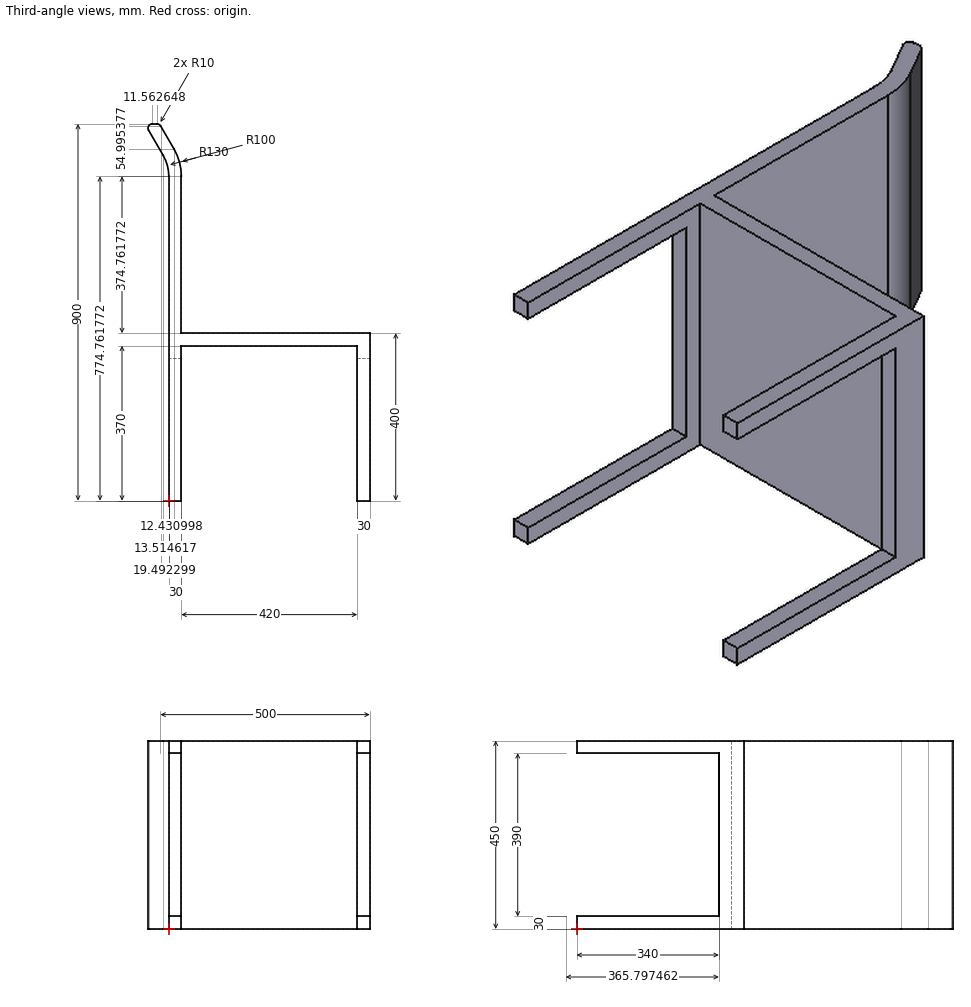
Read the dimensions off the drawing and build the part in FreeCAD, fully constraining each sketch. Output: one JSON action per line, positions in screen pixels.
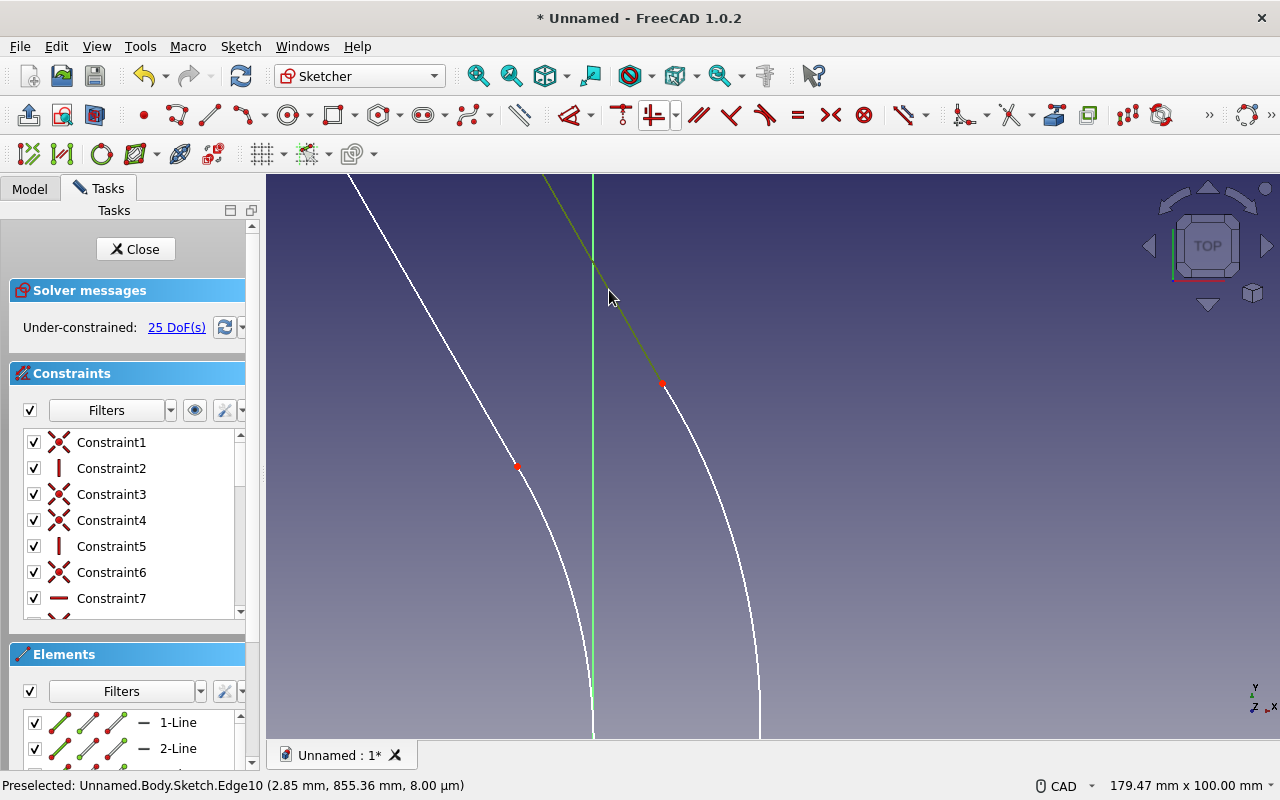
{"action": "scroll", "coordinate": [616, 286], "scroll_direction": "down", "scroll_amount": 13}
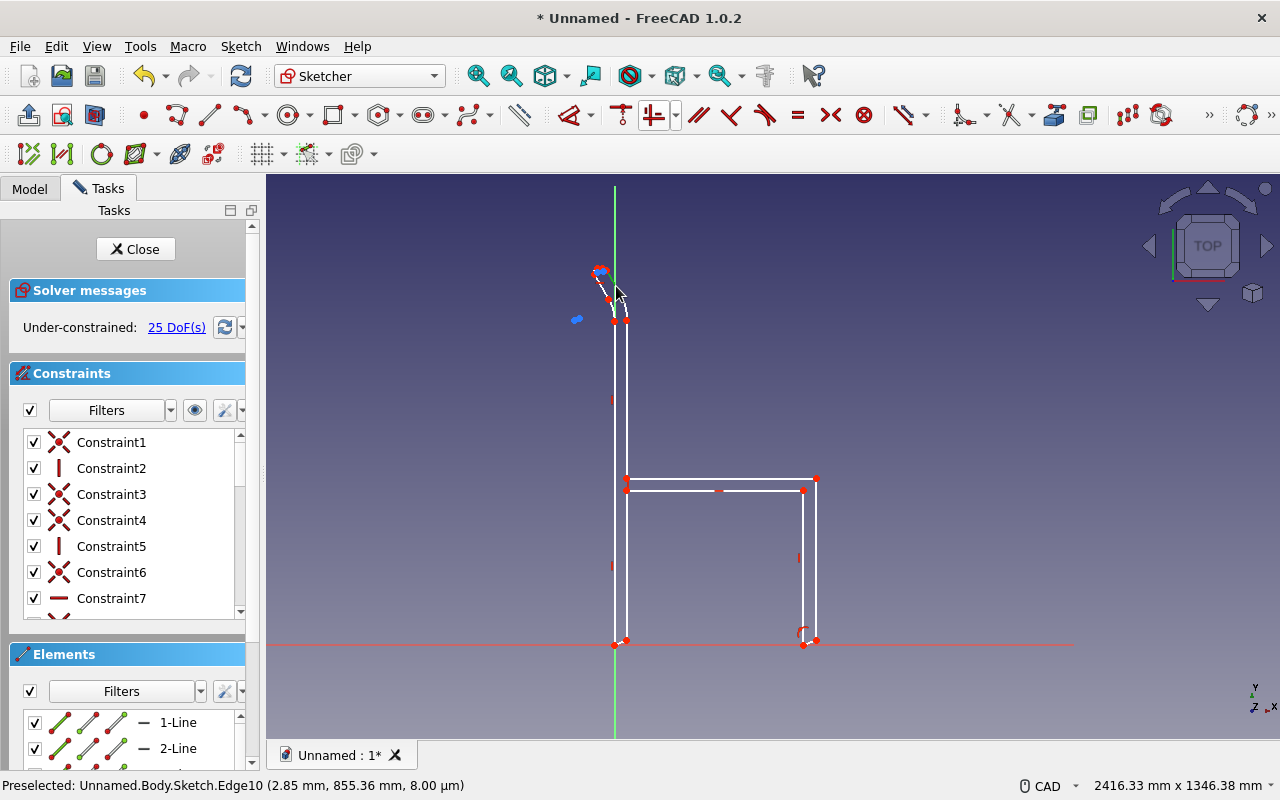
{"action": "scroll", "coordinate": [606, 269], "scroll_direction": "up", "scroll_amount": 12}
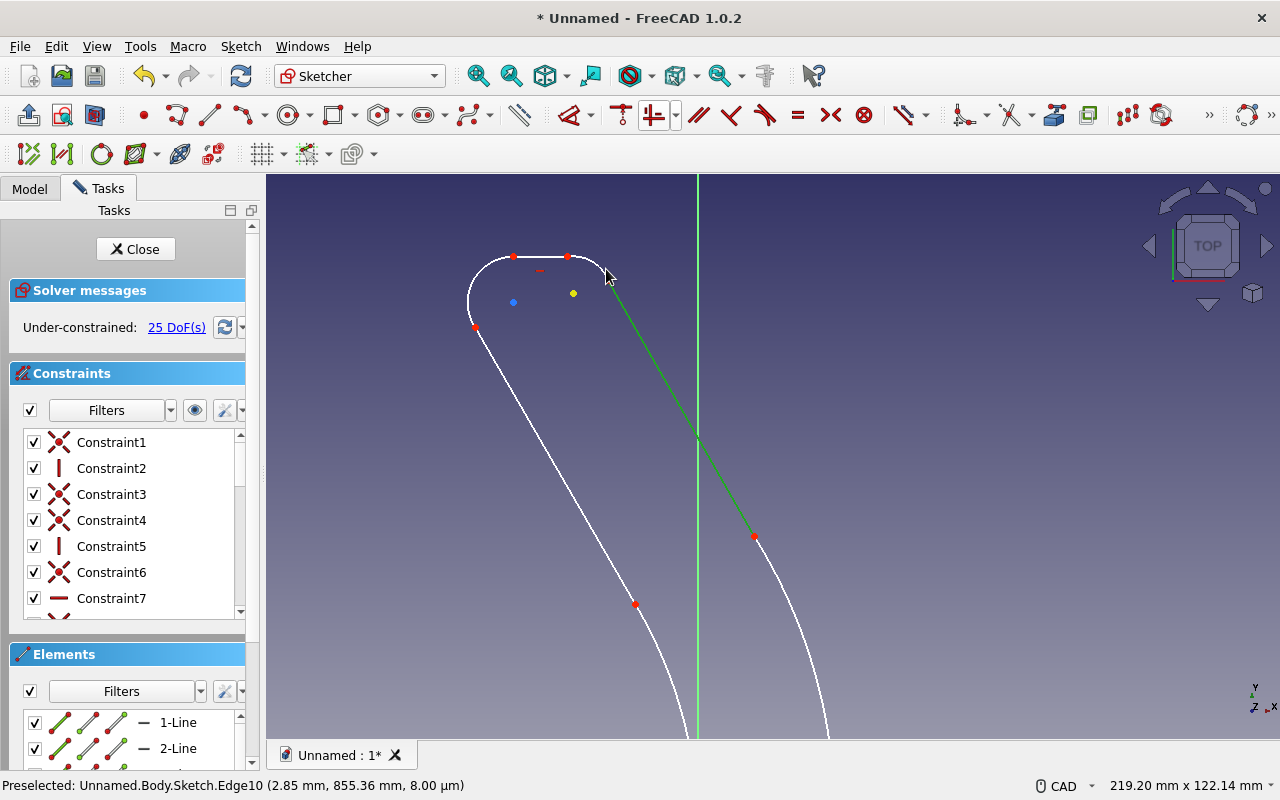
{"action": "left_click", "coordinate": [600, 268]}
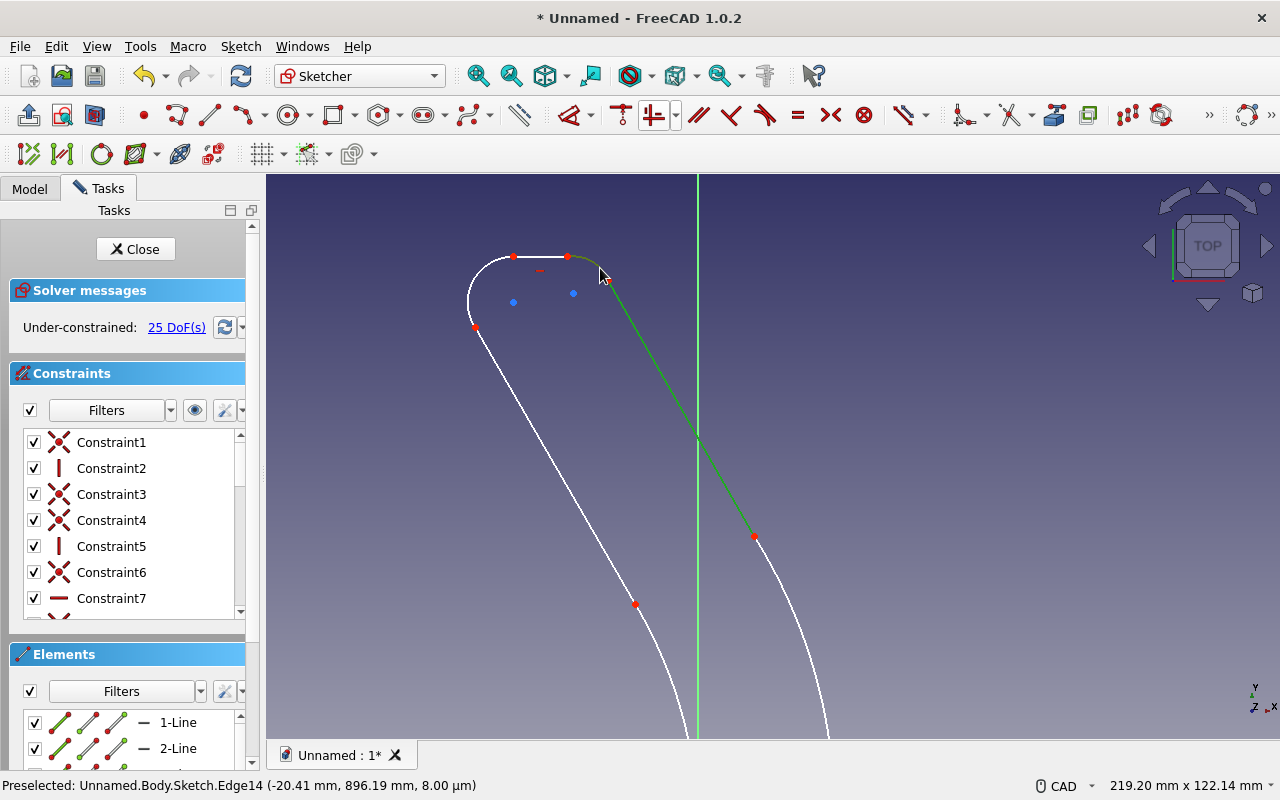
{"action": "left_click", "coordinate": [765, 116]}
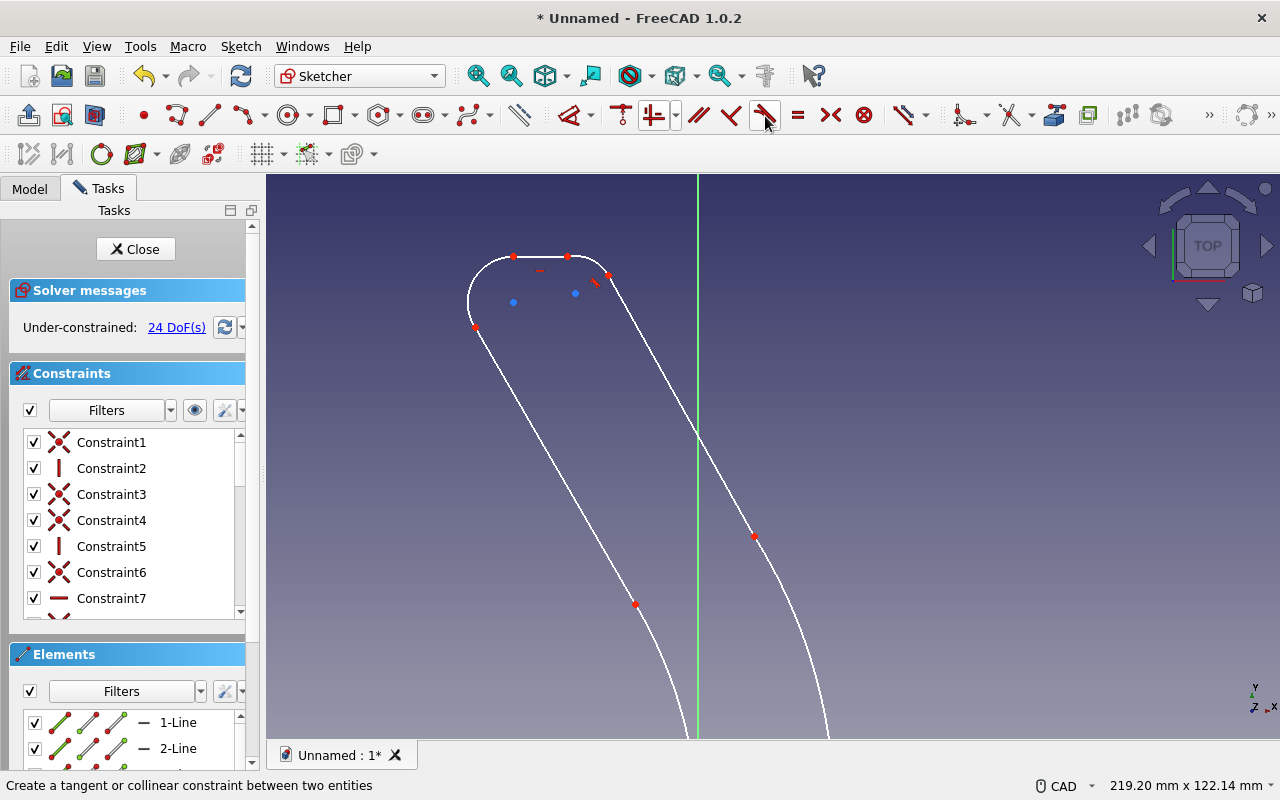
{"action": "left_click", "coordinate": [551, 257]}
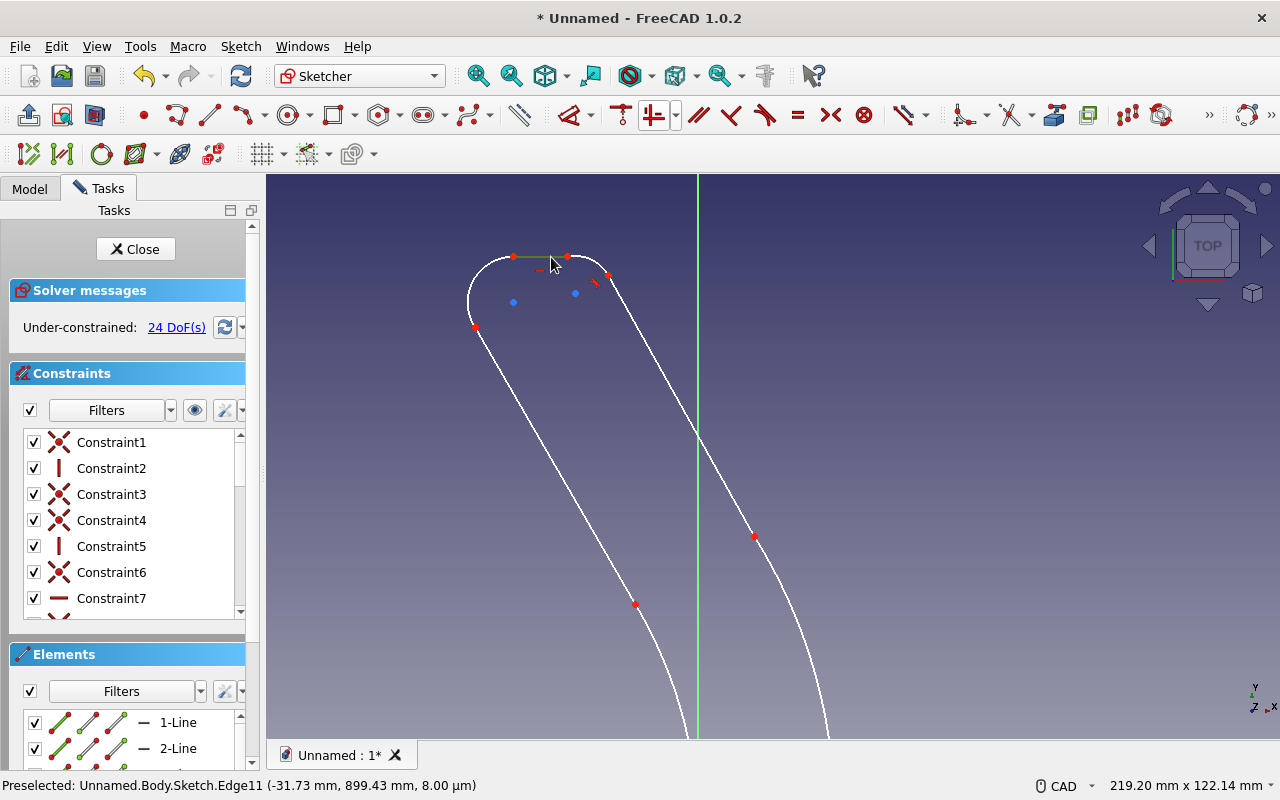
{"action": "left_click", "coordinate": [599, 264]}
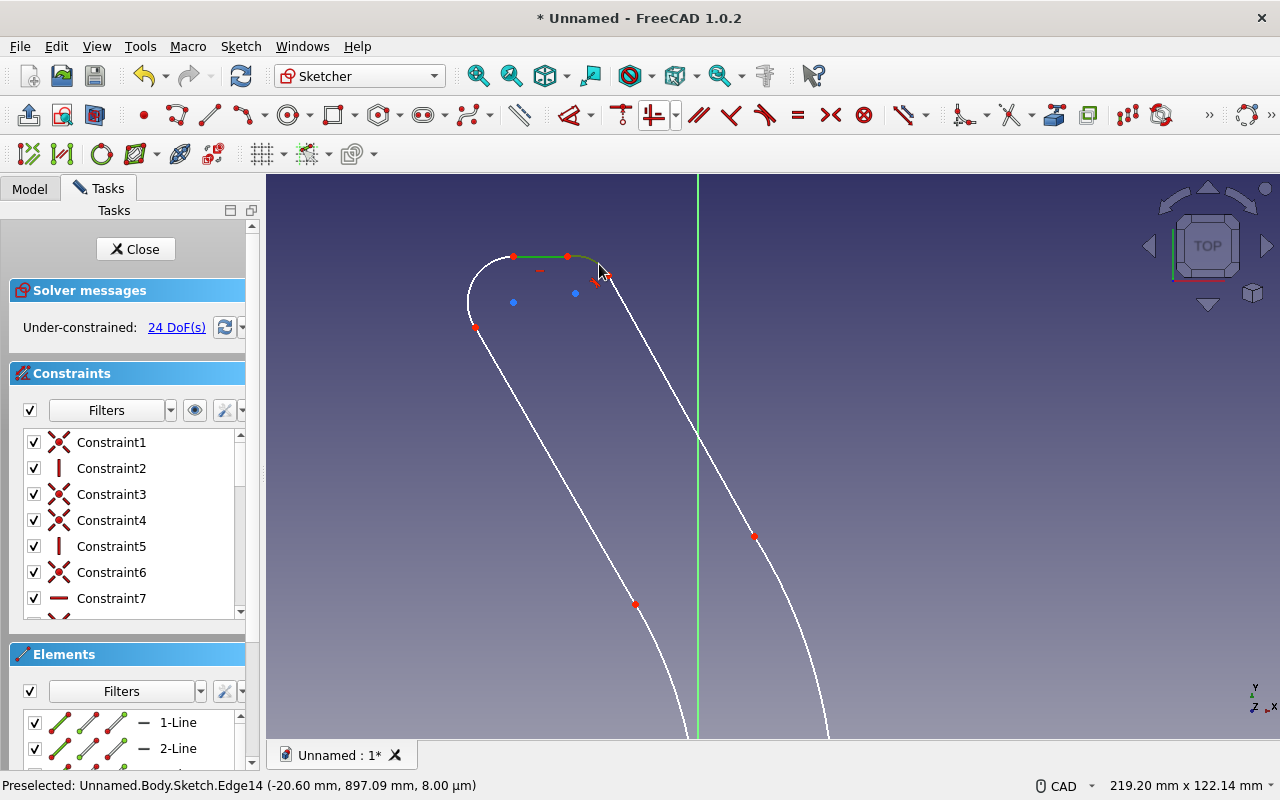
{"action": "left_click", "coordinate": [765, 116]}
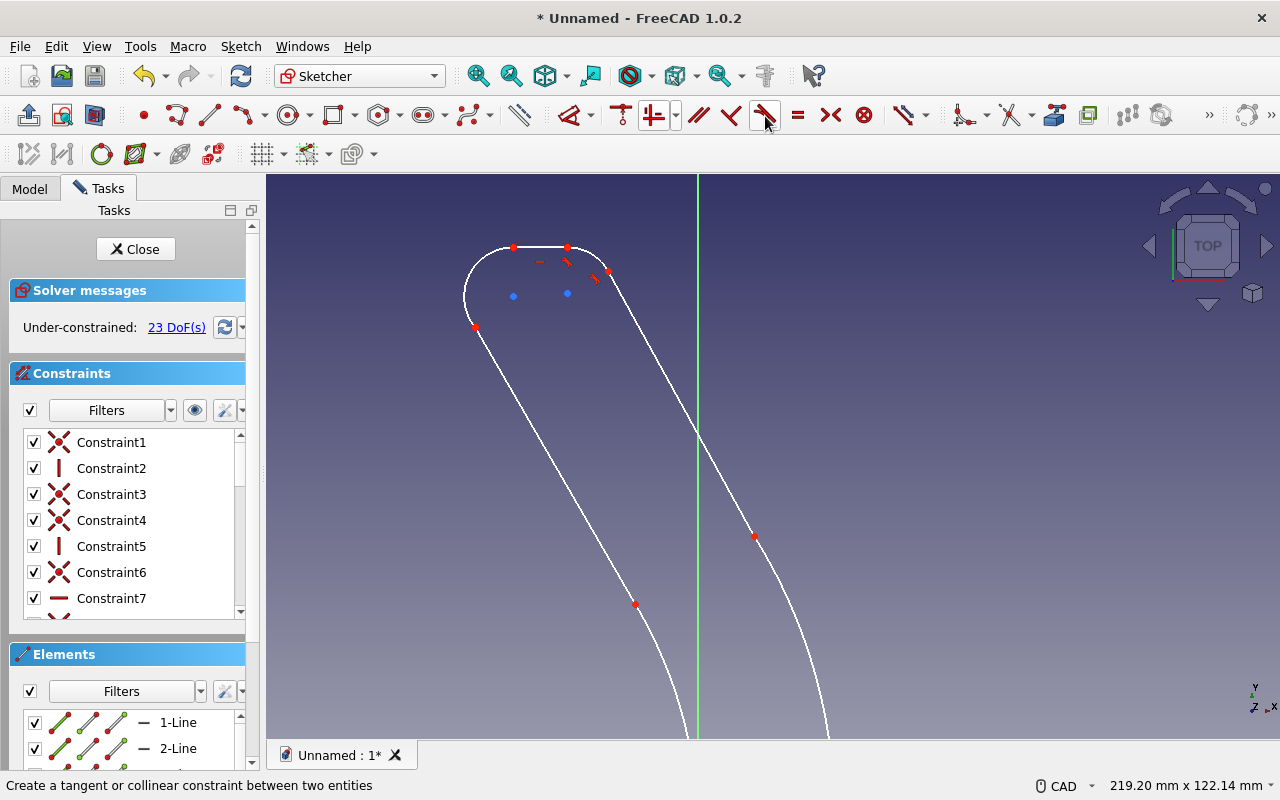
{"action": "left_click", "coordinate": [551, 247]}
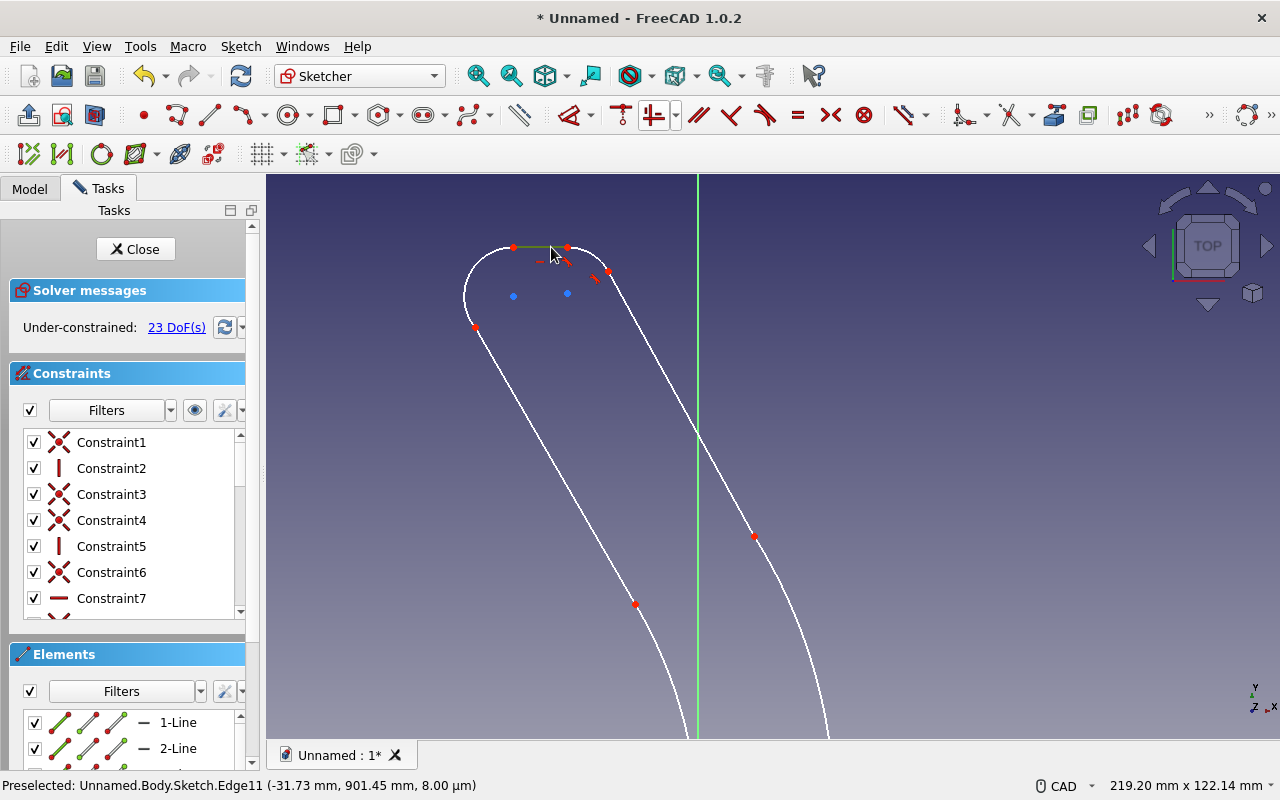
{"action": "left_click", "coordinate": [483, 258]}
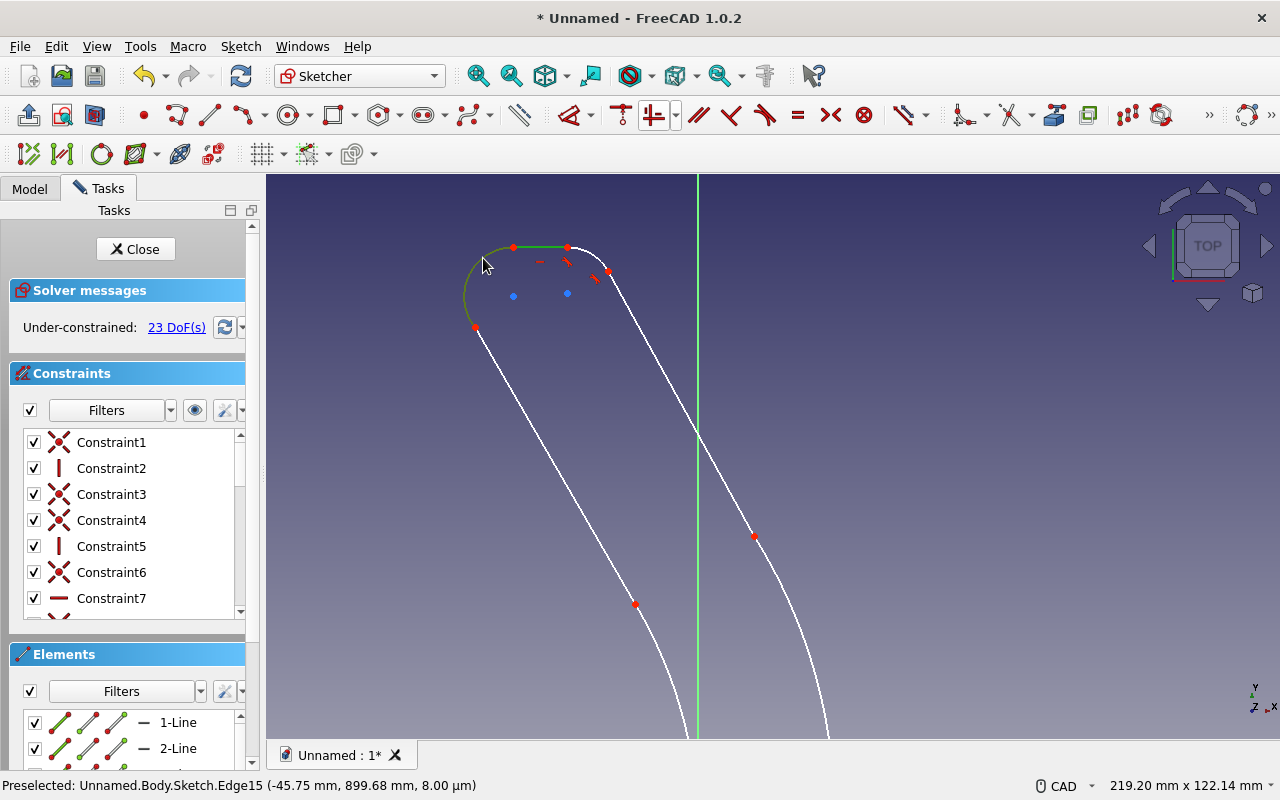
{"action": "left_click", "coordinate": [765, 116]}